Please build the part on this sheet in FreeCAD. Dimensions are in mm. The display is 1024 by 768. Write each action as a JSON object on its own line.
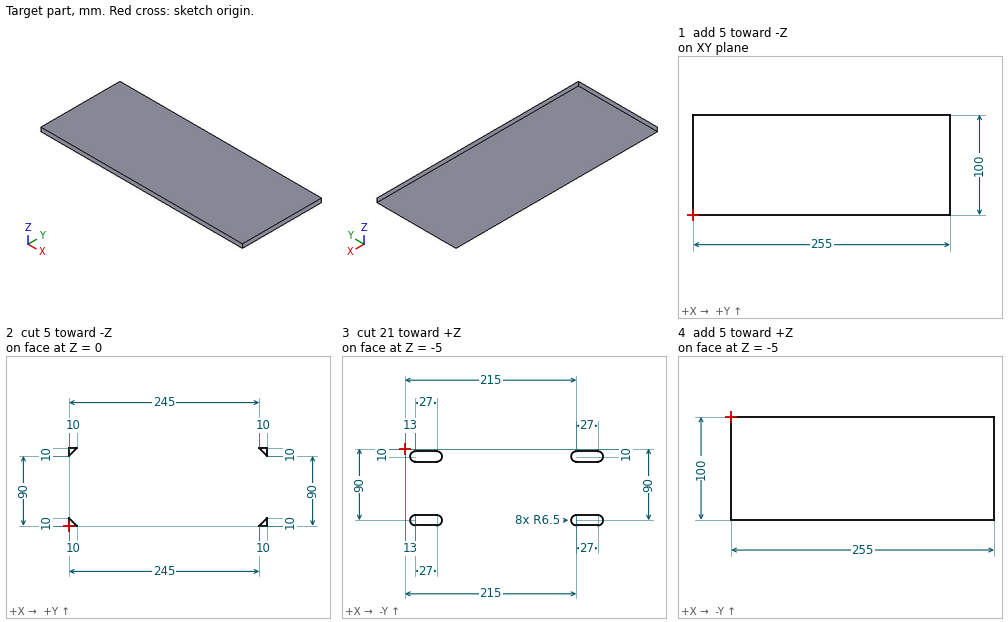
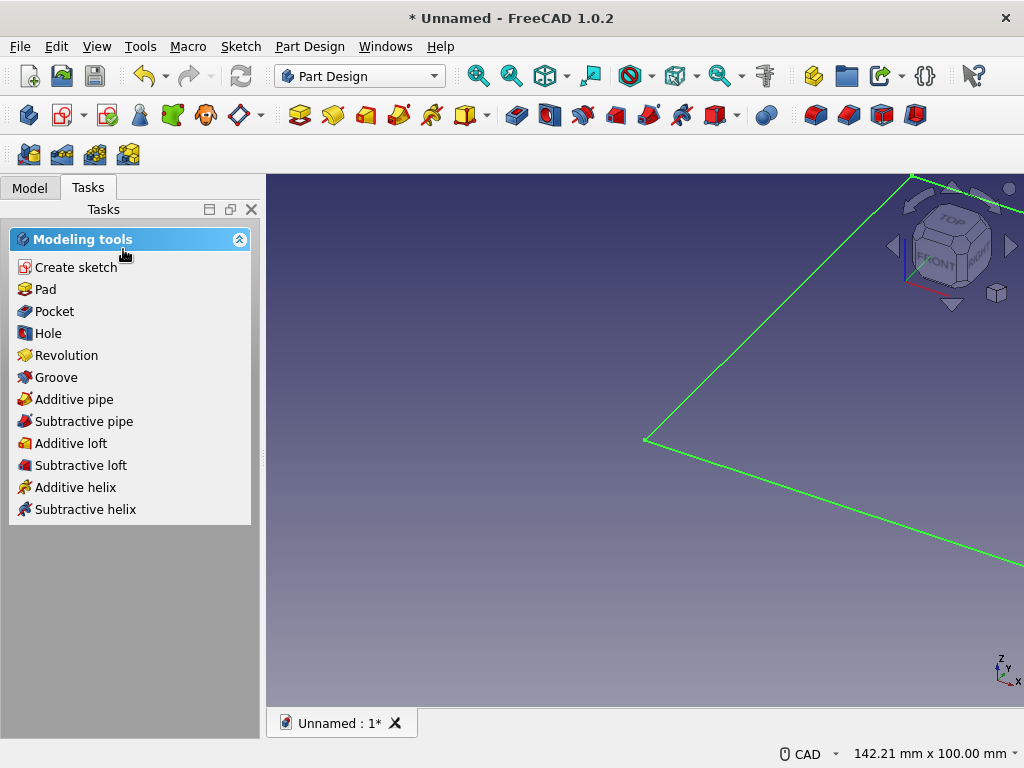
{"action": "left_click", "coordinate": [300, 116]}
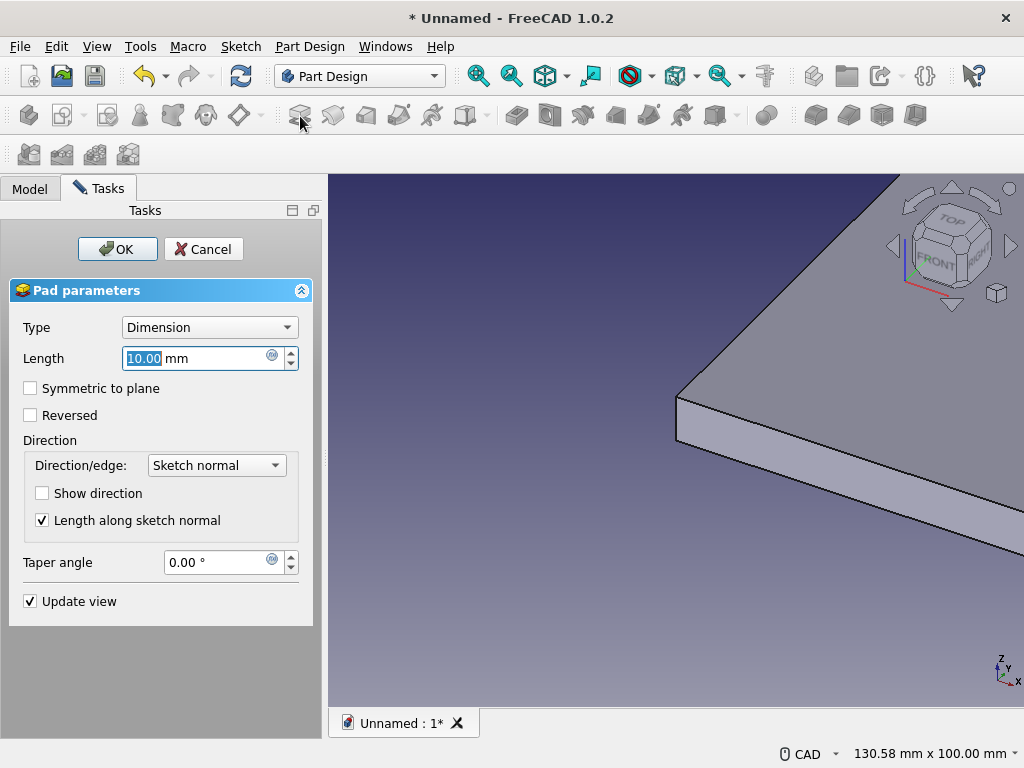
{"action": "type", "text": "5"}
{"action": "key", "text": "Tab"}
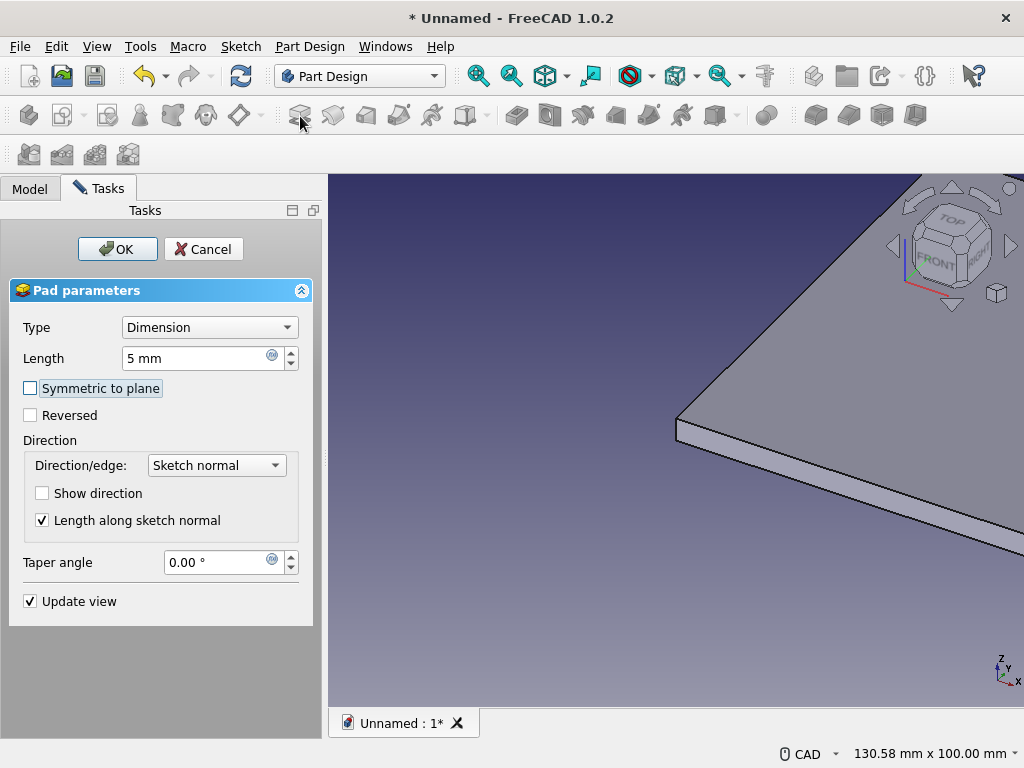
{"action": "left_click", "coordinate": [31, 415]}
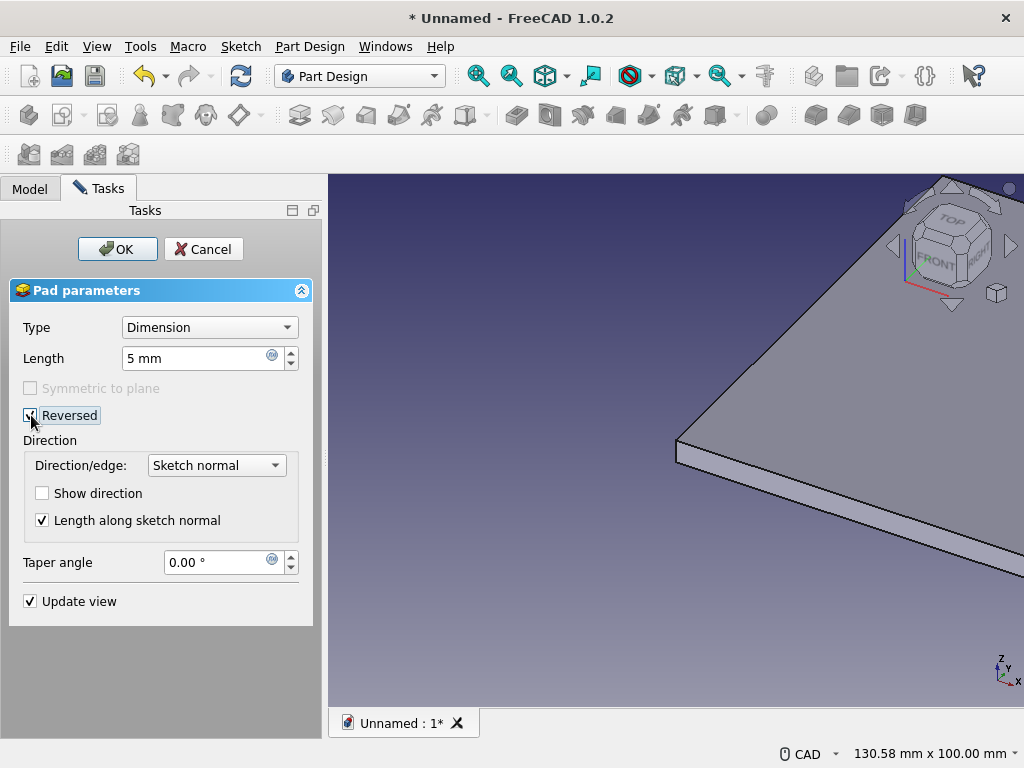
{"action": "left_click", "coordinate": [118, 249]}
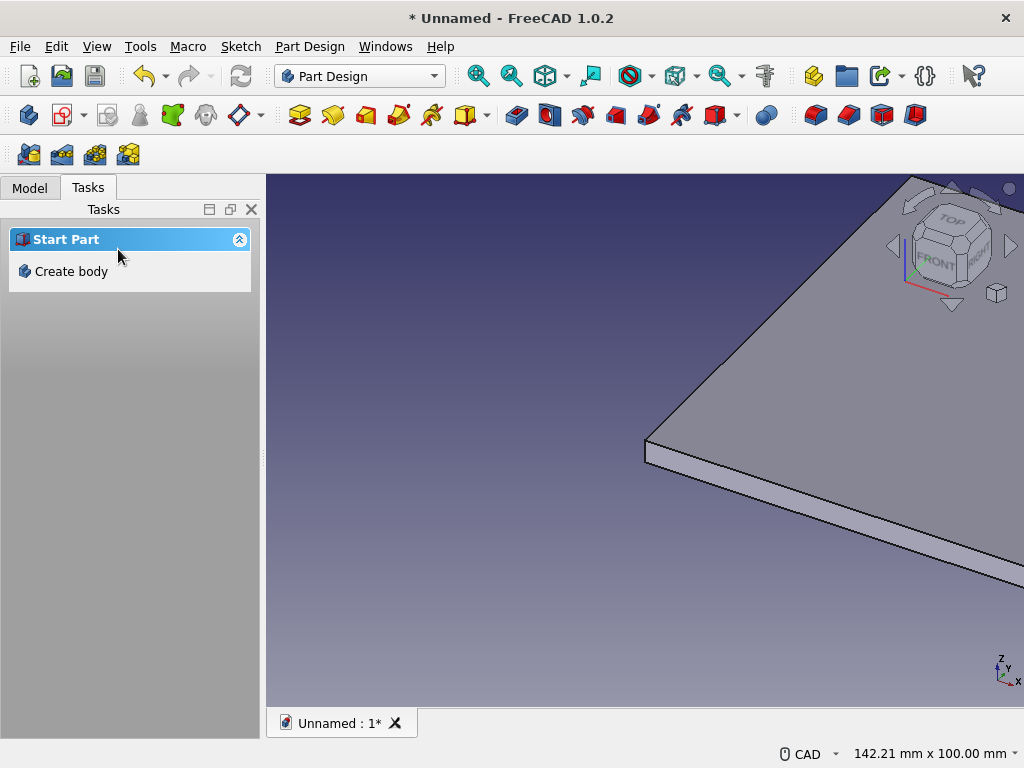
{"action": "key", "text": "v f"}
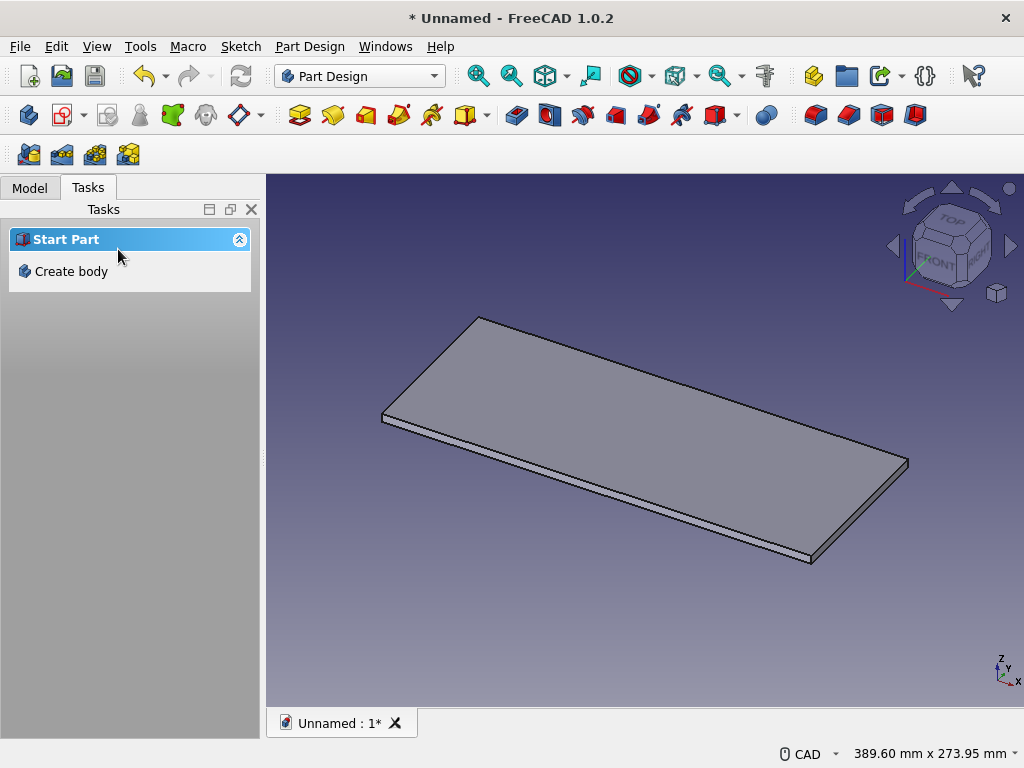
{"action": "left_click", "coordinate": [768, 476]}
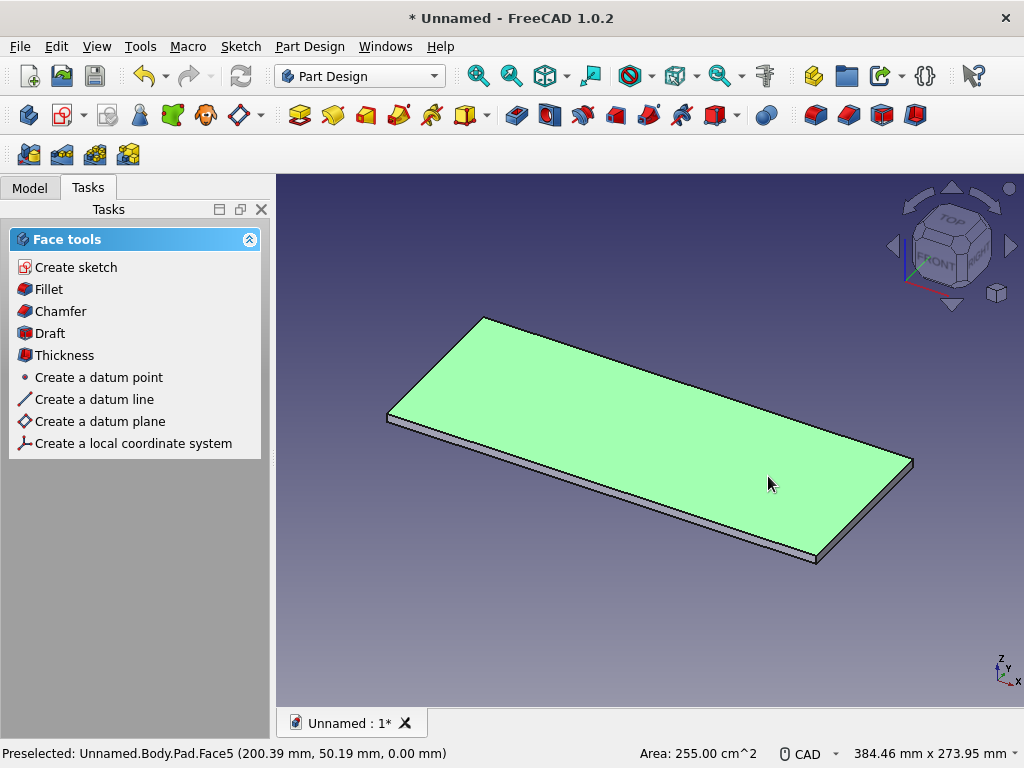
{"action": "left_click", "coordinate": [62, 116]}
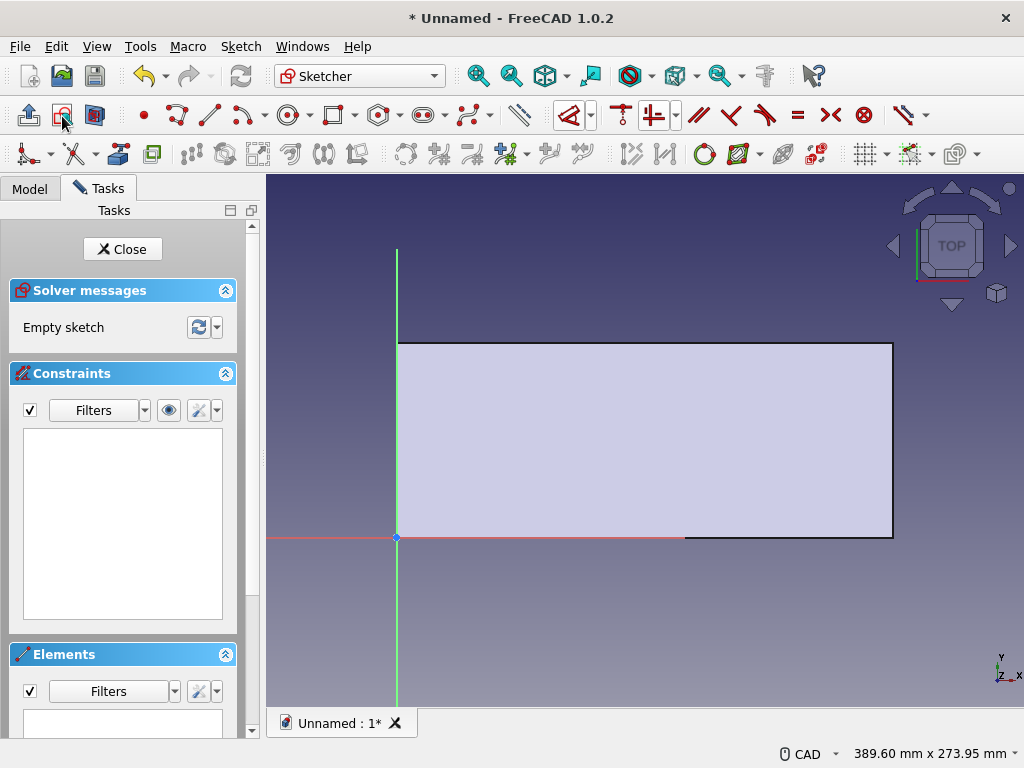
{"action": "scroll", "coordinate": [294, 441], "scroll_direction": "down", "scroll_amount": 1}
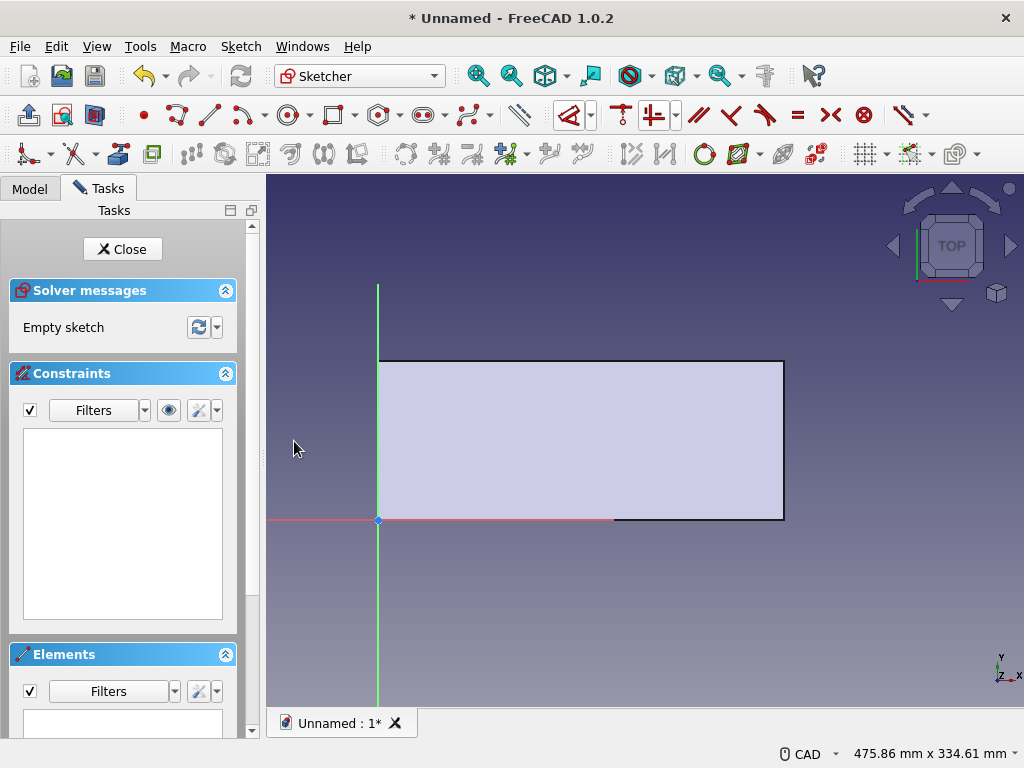
{"action": "left_click", "coordinate": [177, 116]}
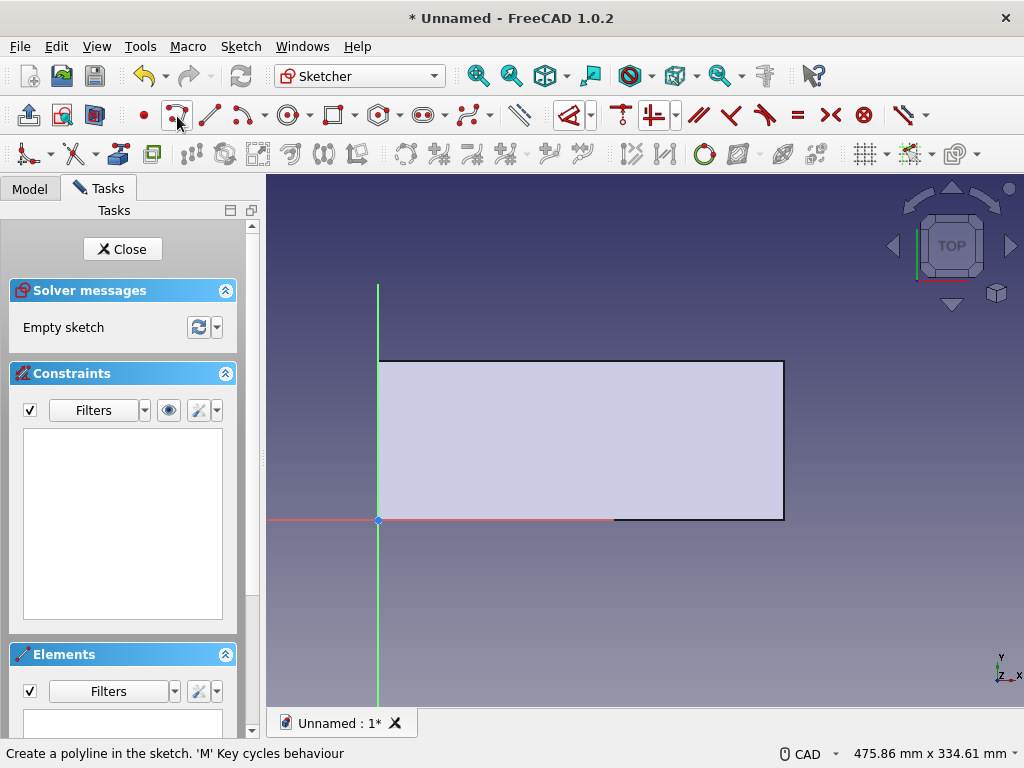
{"action": "left_click", "coordinate": [378, 377]}
{"action": "left_click", "coordinate": [394, 361]}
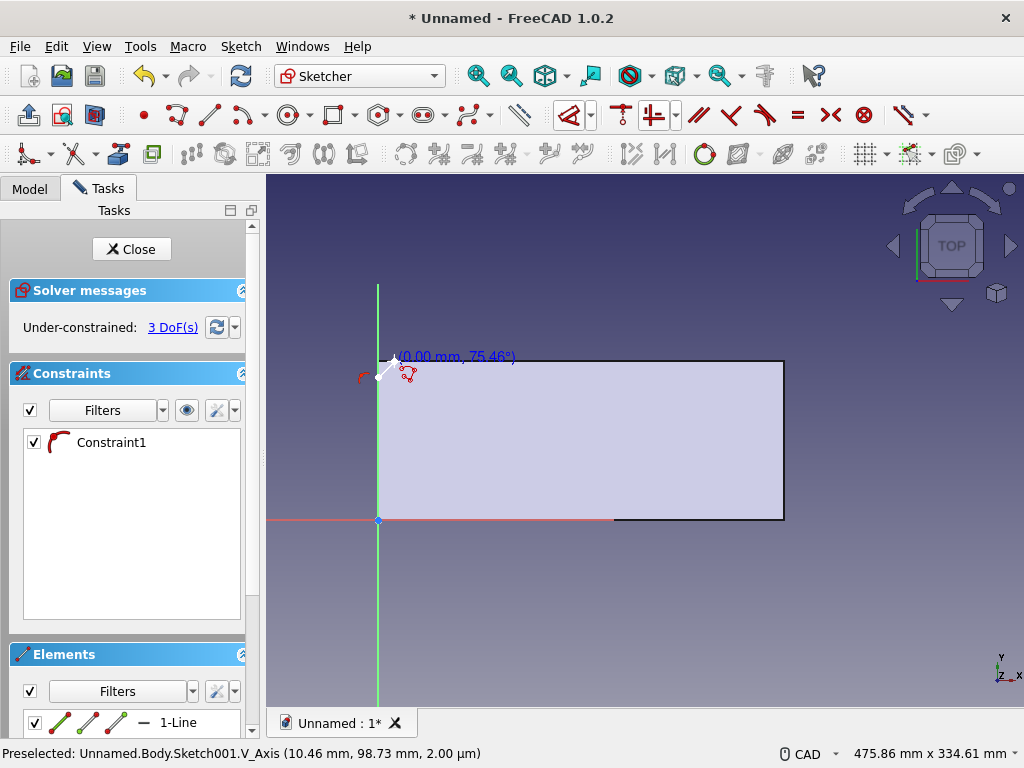
{"action": "scroll", "coordinate": [378, 361], "scroll_direction": "up", "scroll_amount": 2}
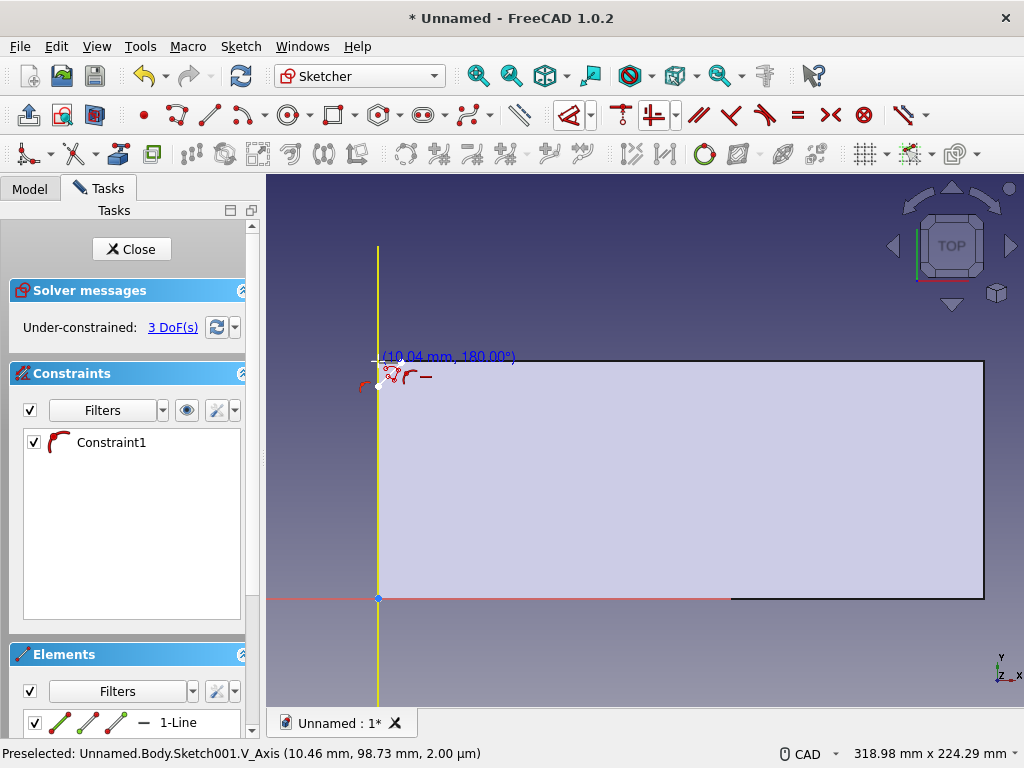
{"action": "left_click", "coordinate": [387, 361]}
{"action": "left_click", "coordinate": [378, 386]}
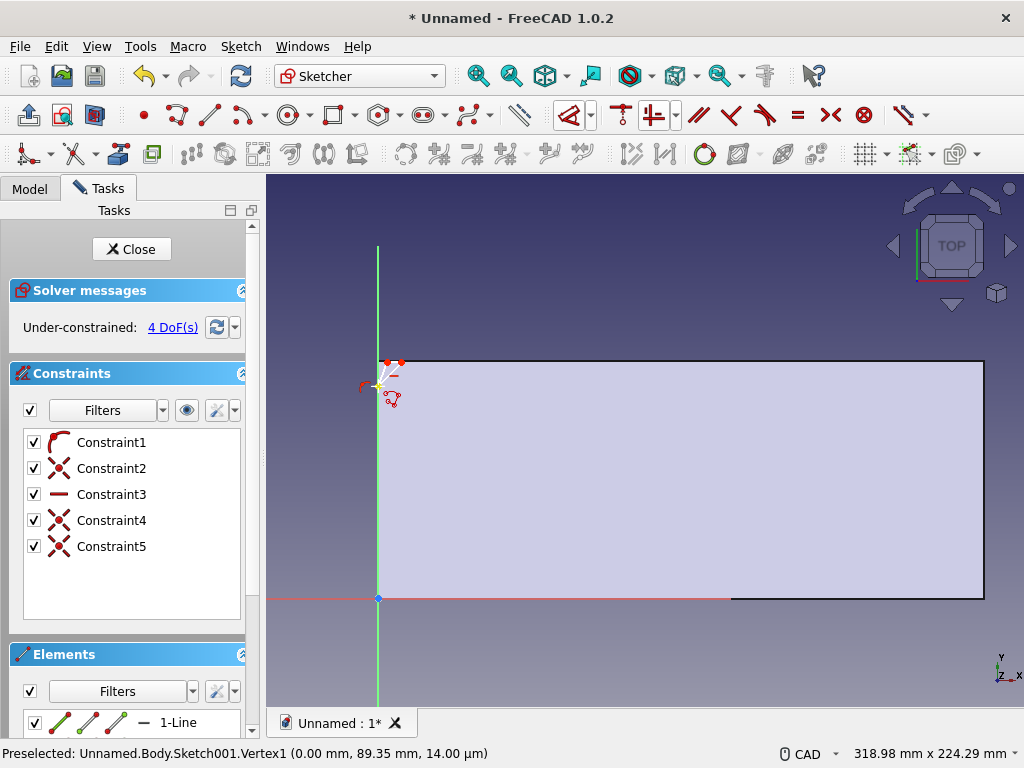
{"action": "scroll", "coordinate": [363, 361], "scroll_direction": "down", "scroll_amount": 2}